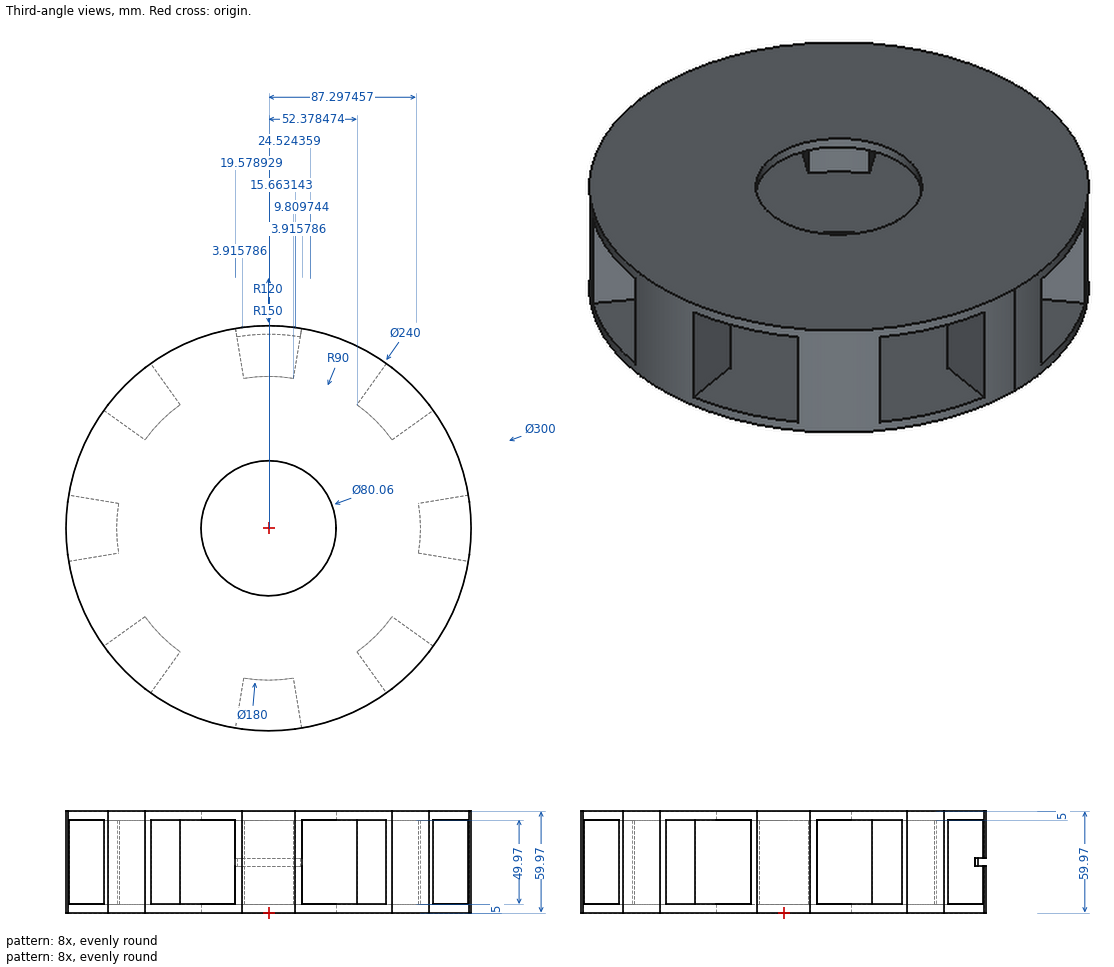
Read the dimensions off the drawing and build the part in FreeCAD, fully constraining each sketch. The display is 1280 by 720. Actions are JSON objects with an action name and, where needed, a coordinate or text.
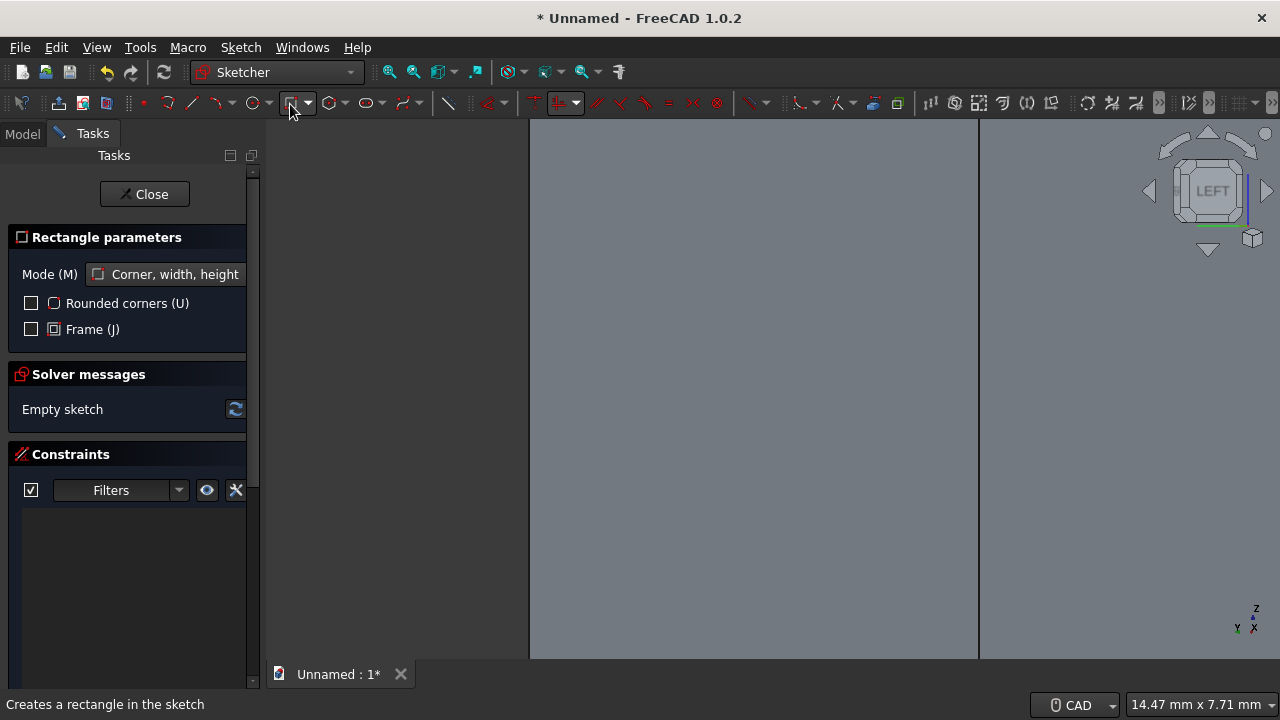
{"action": "left_click", "coordinate": [529, 213]}
{"action": "left_click", "coordinate": [880, 563]}
{"action": "key", "text": "Escape"}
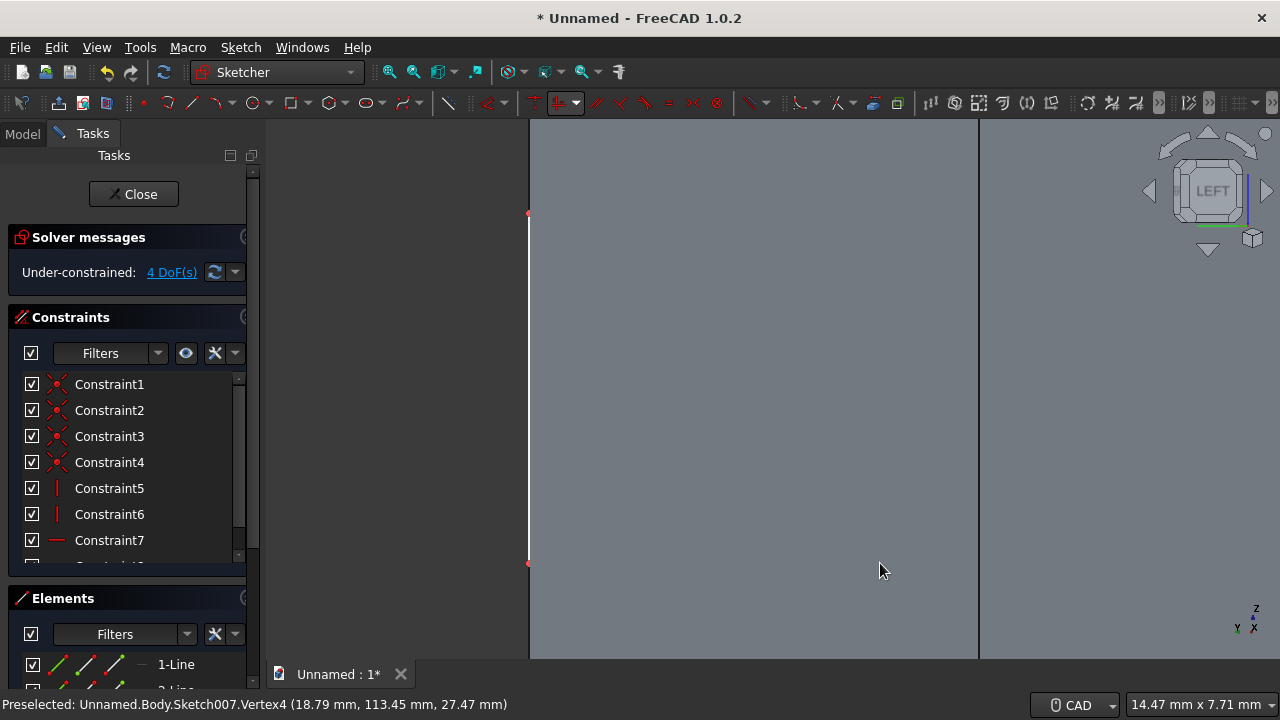
{"action": "key", "text": "d"}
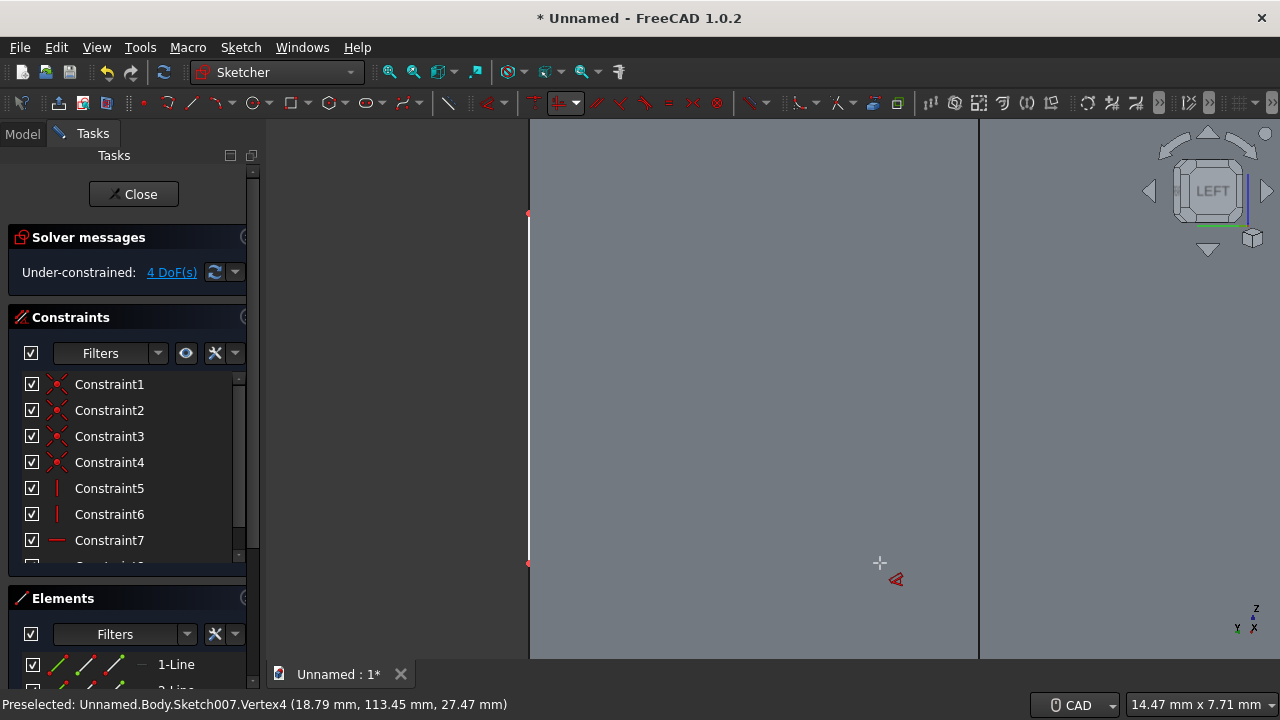
{"action": "left_click", "coordinate": [529, 319]}
{"action": "left_click", "coordinate": [495, 389]}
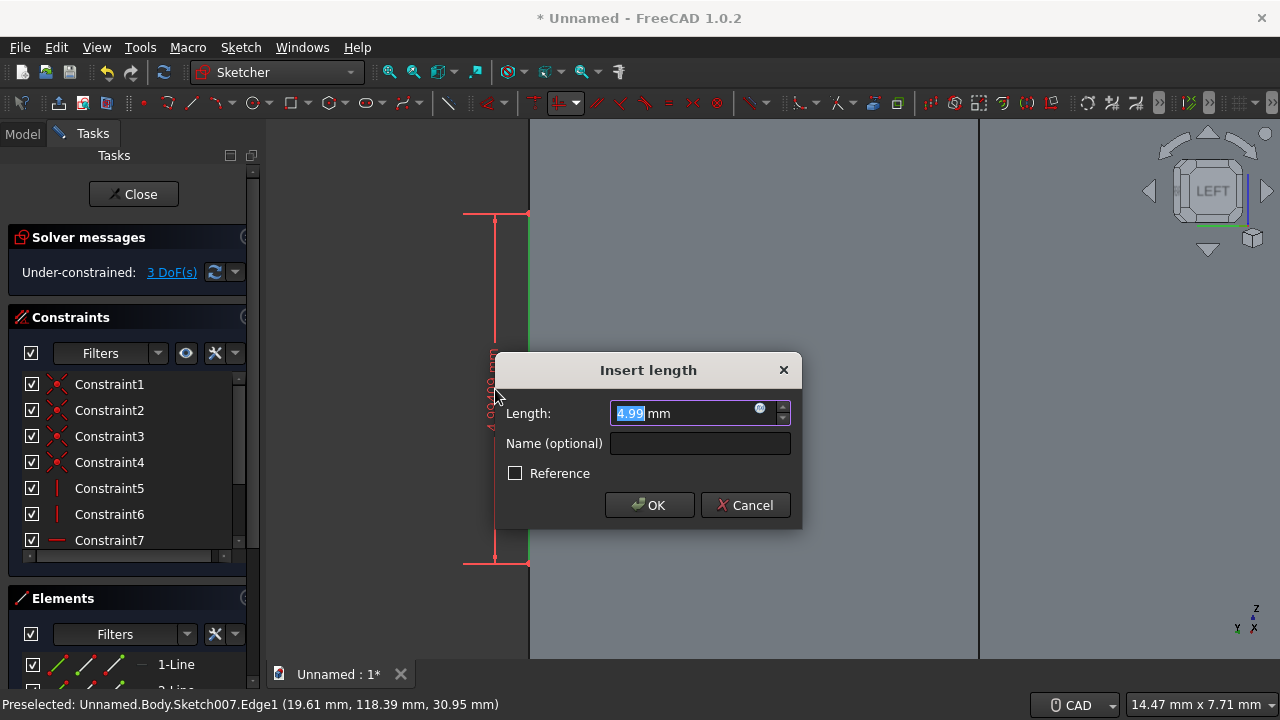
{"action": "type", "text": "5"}
{"action": "key", "text": "Return"}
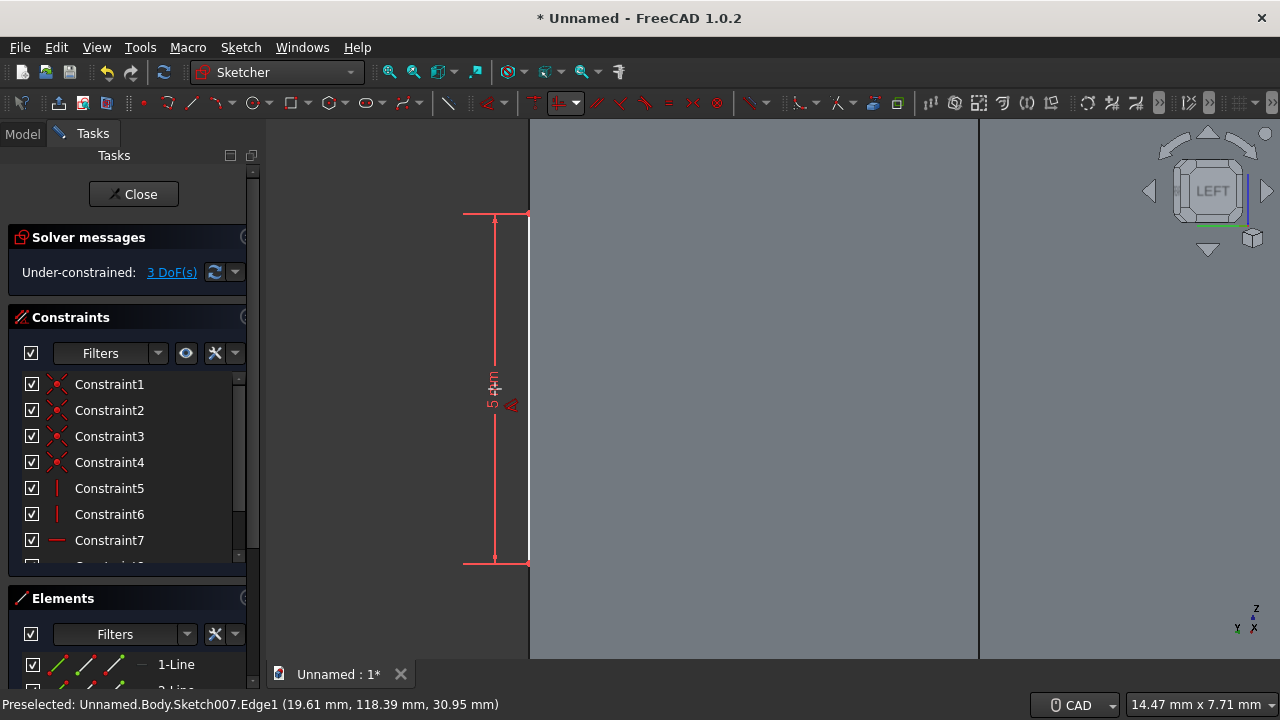
{"action": "left_click", "coordinate": [634, 564]}
{"action": "left_click", "coordinate": [704, 598]}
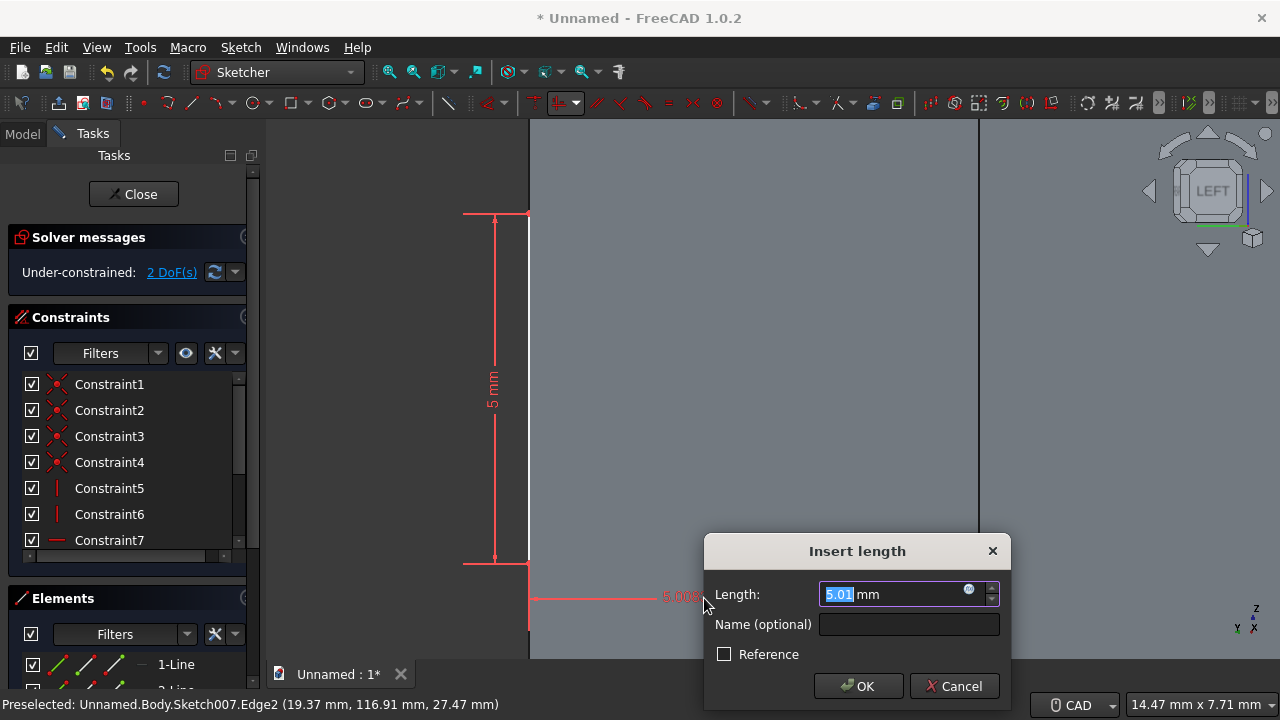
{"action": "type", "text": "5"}
{"action": "key", "text": "Return"}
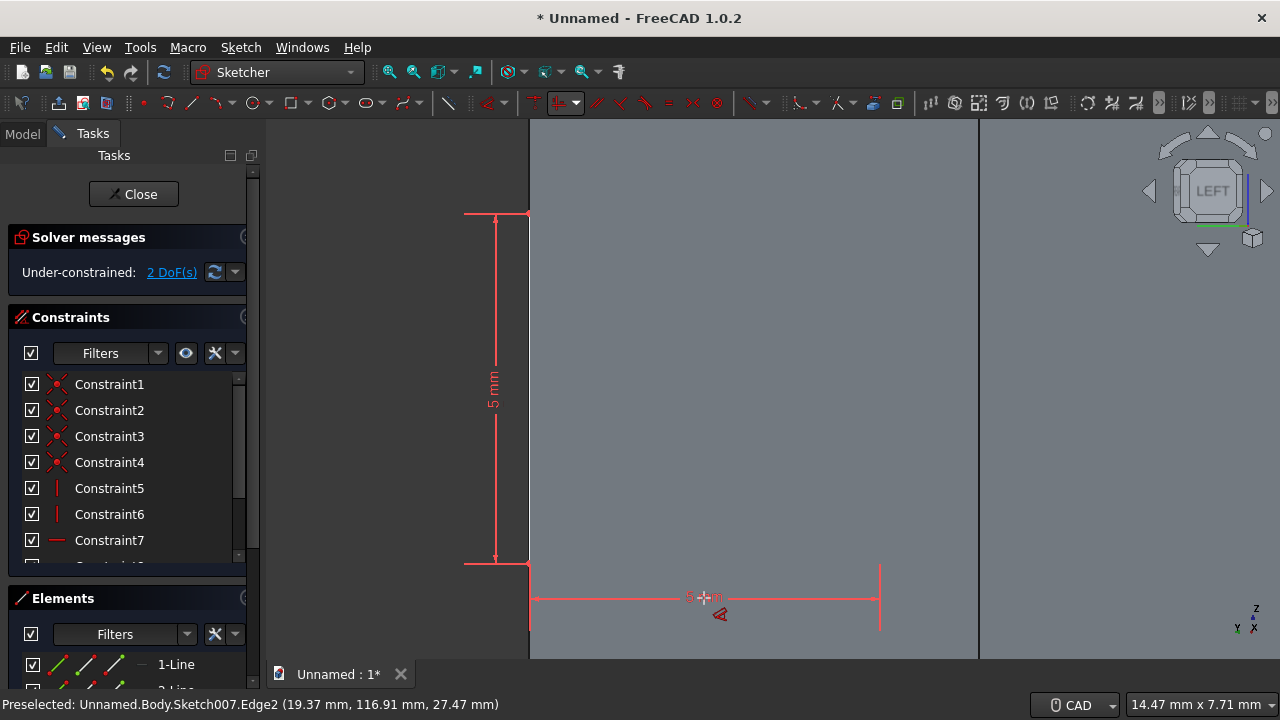
{"action": "left_click", "coordinate": [530, 214]}
{"action": "left_click", "coordinate": [822, 180]}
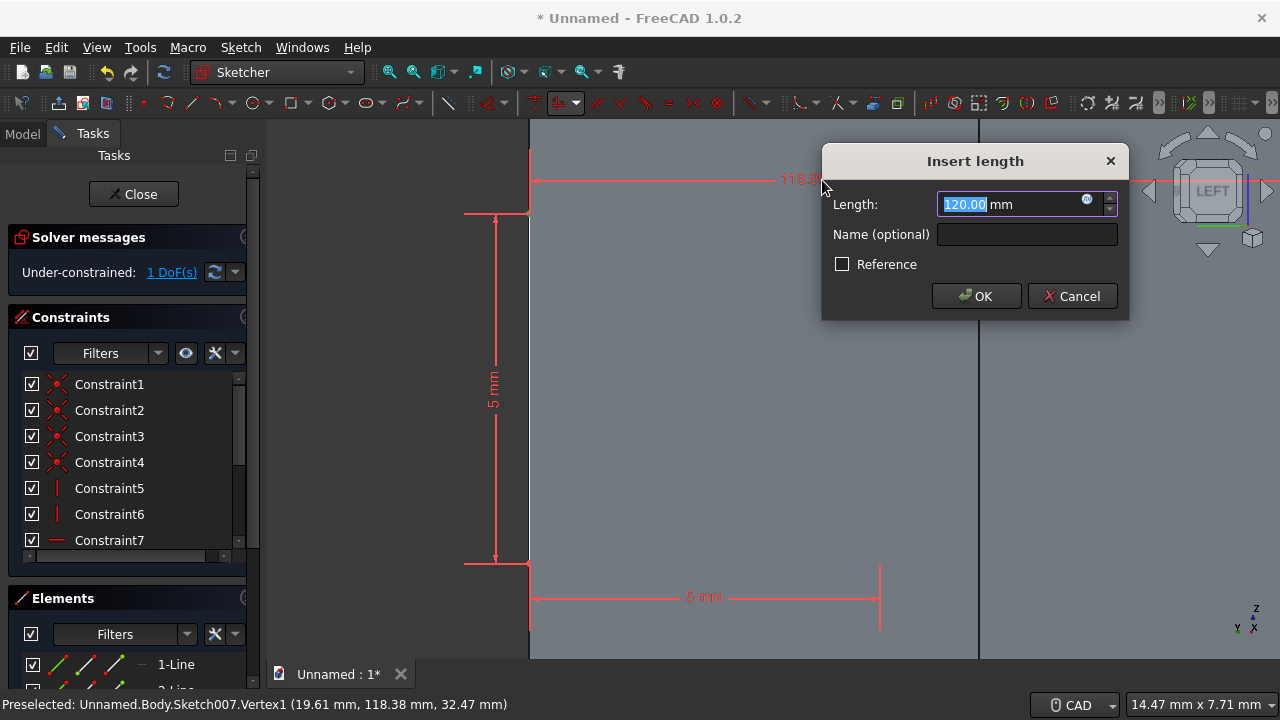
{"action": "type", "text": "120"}
{"action": "key", "text": "Return"}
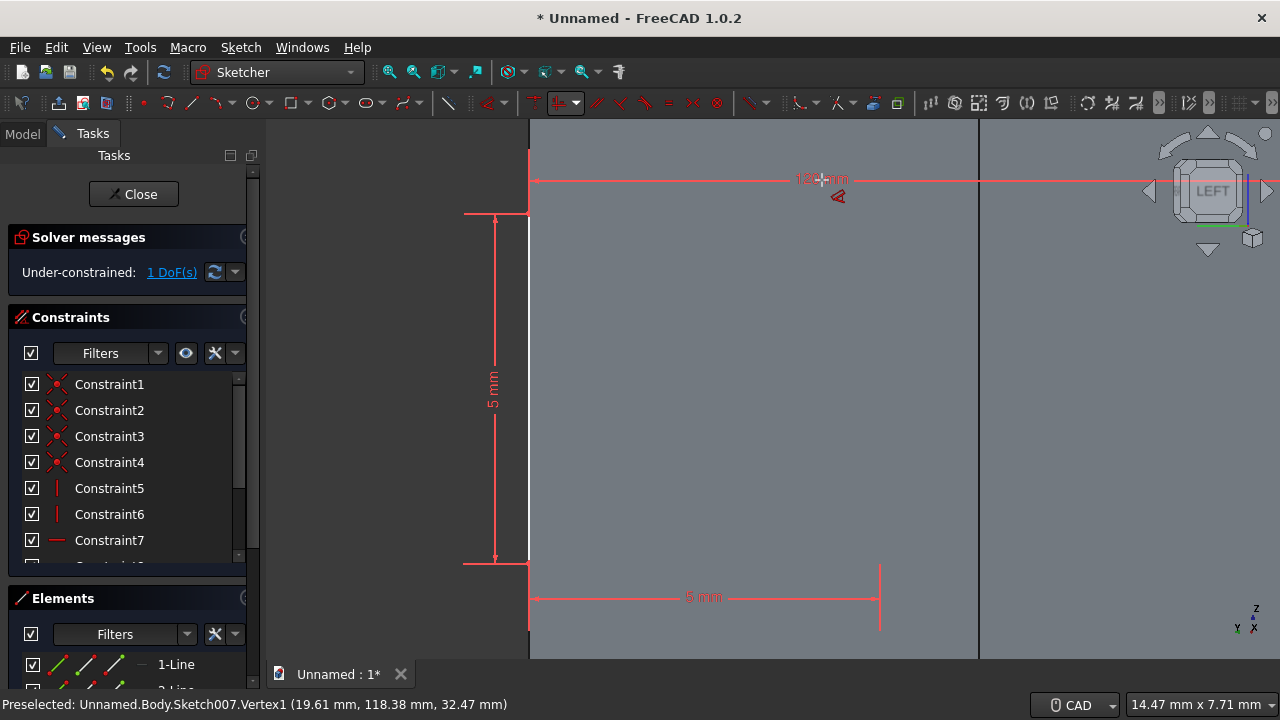
{"action": "left_click", "coordinate": [529, 214]}
{"action": "left_click", "coordinate": [495, 422]}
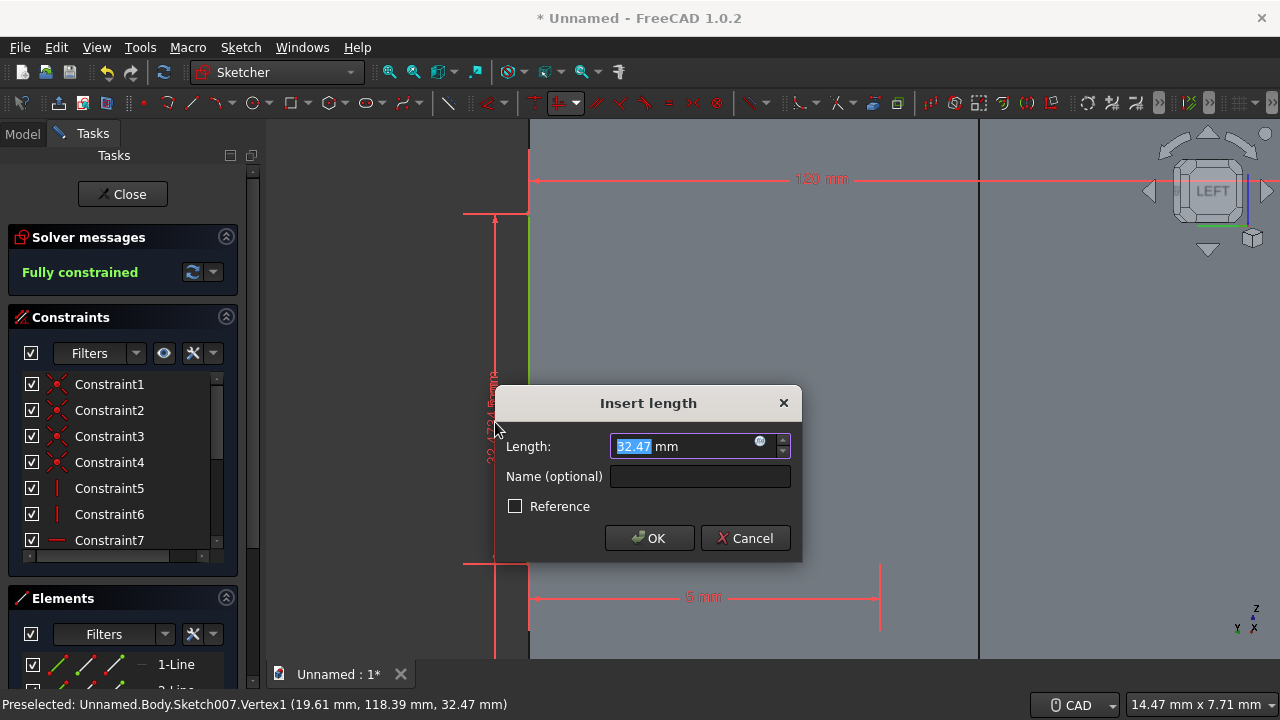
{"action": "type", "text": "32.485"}
{"action": "key", "text": "Return"}
{"action": "key", "text": "Escape"}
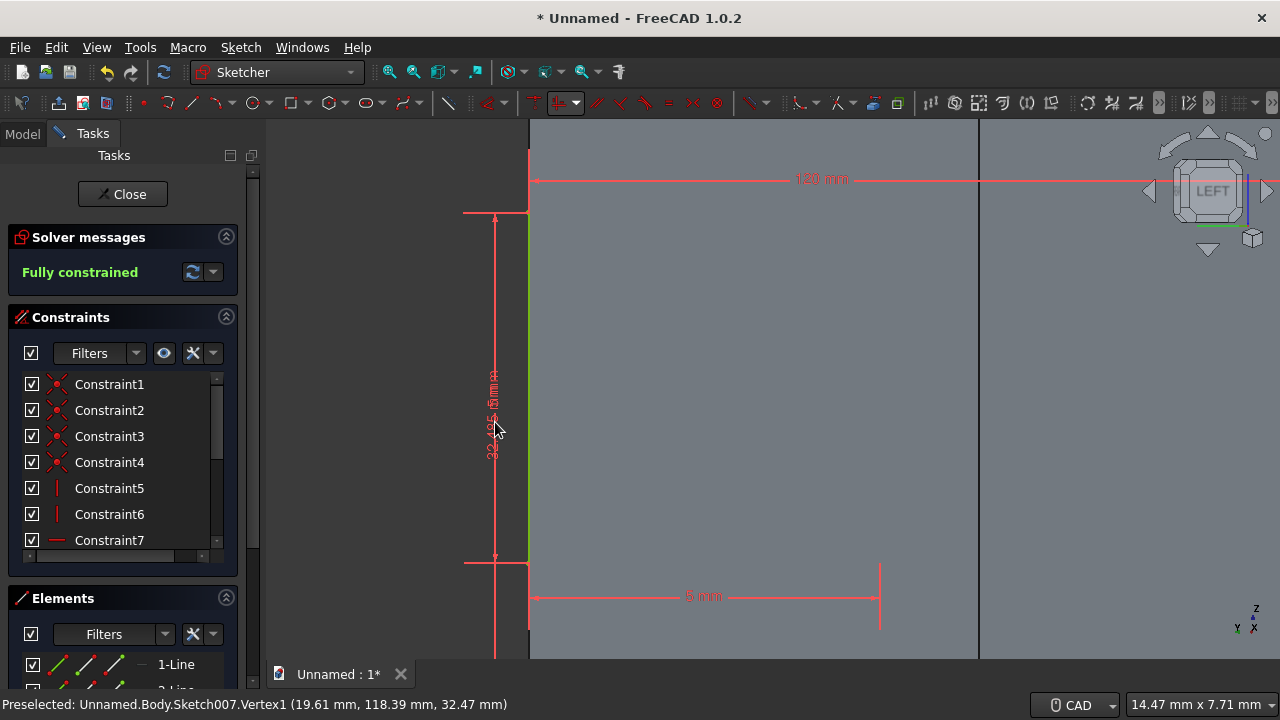
{"action": "left_click", "coordinate": [123, 194]}